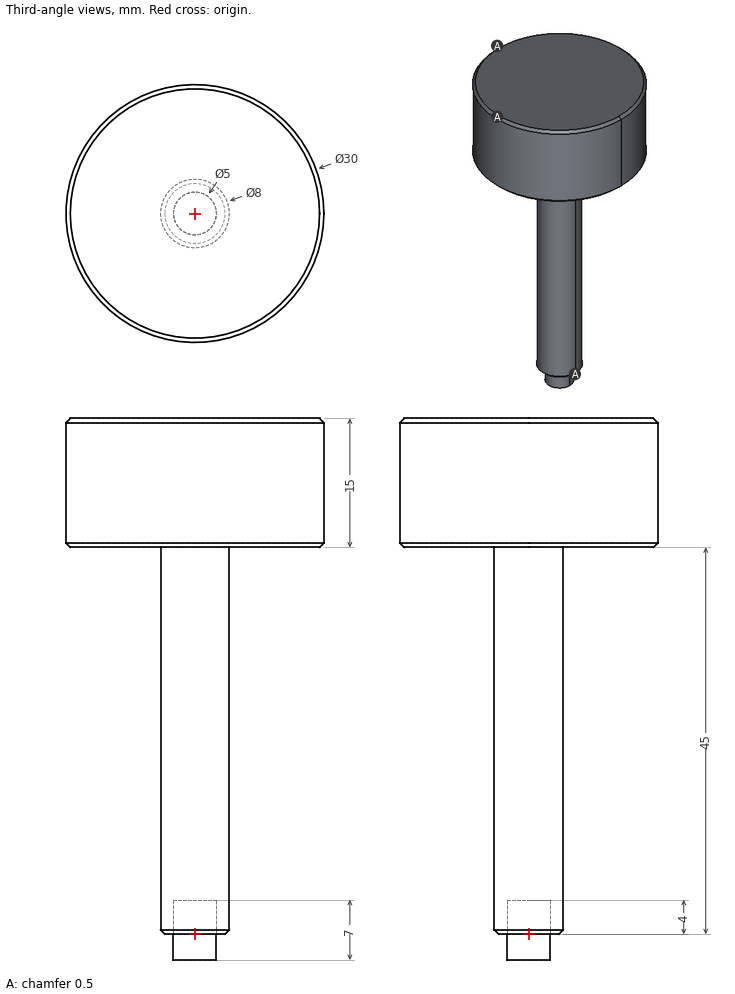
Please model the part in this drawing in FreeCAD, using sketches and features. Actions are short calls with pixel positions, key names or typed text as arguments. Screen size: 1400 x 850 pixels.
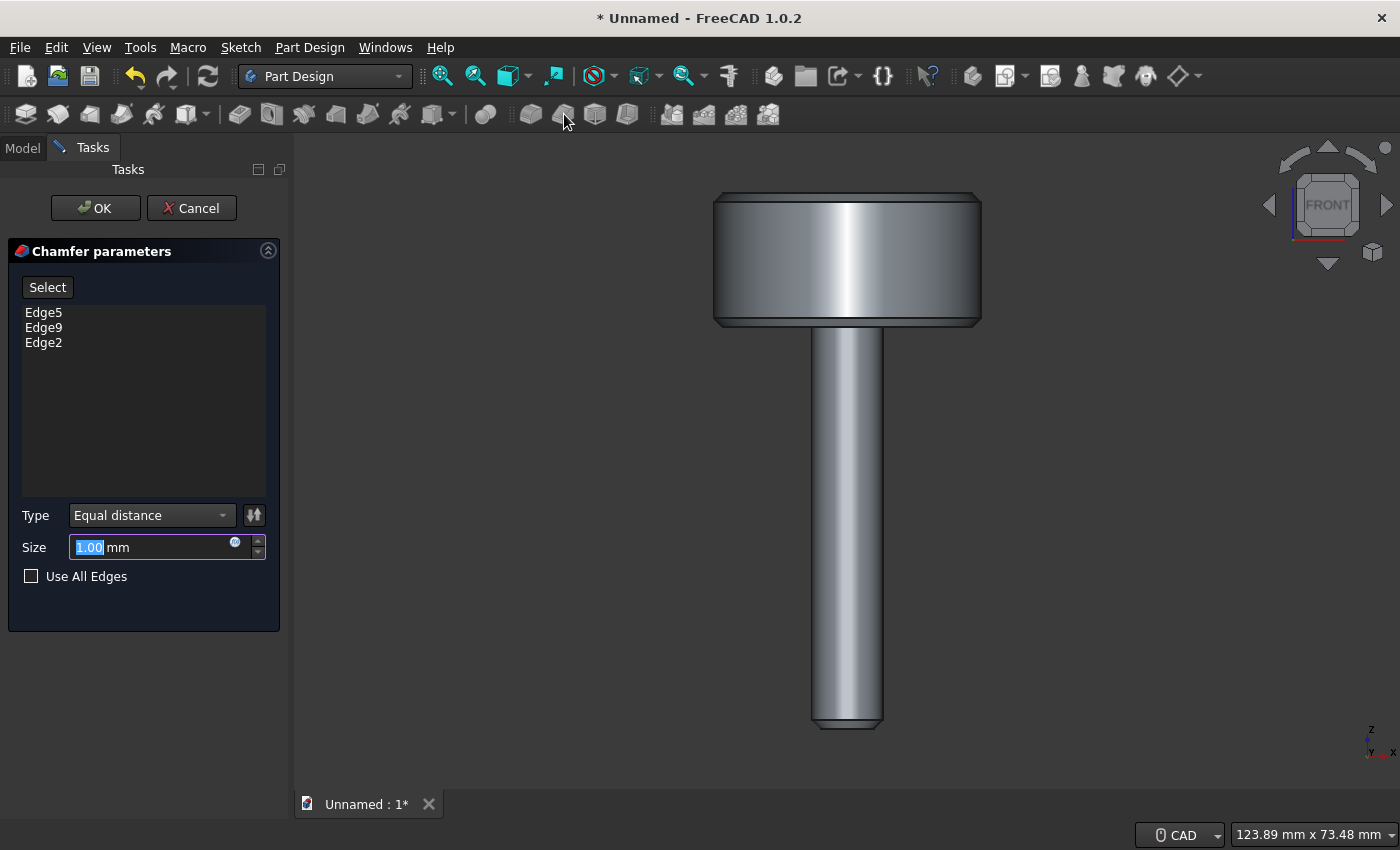
text(0.5)
key(Tab)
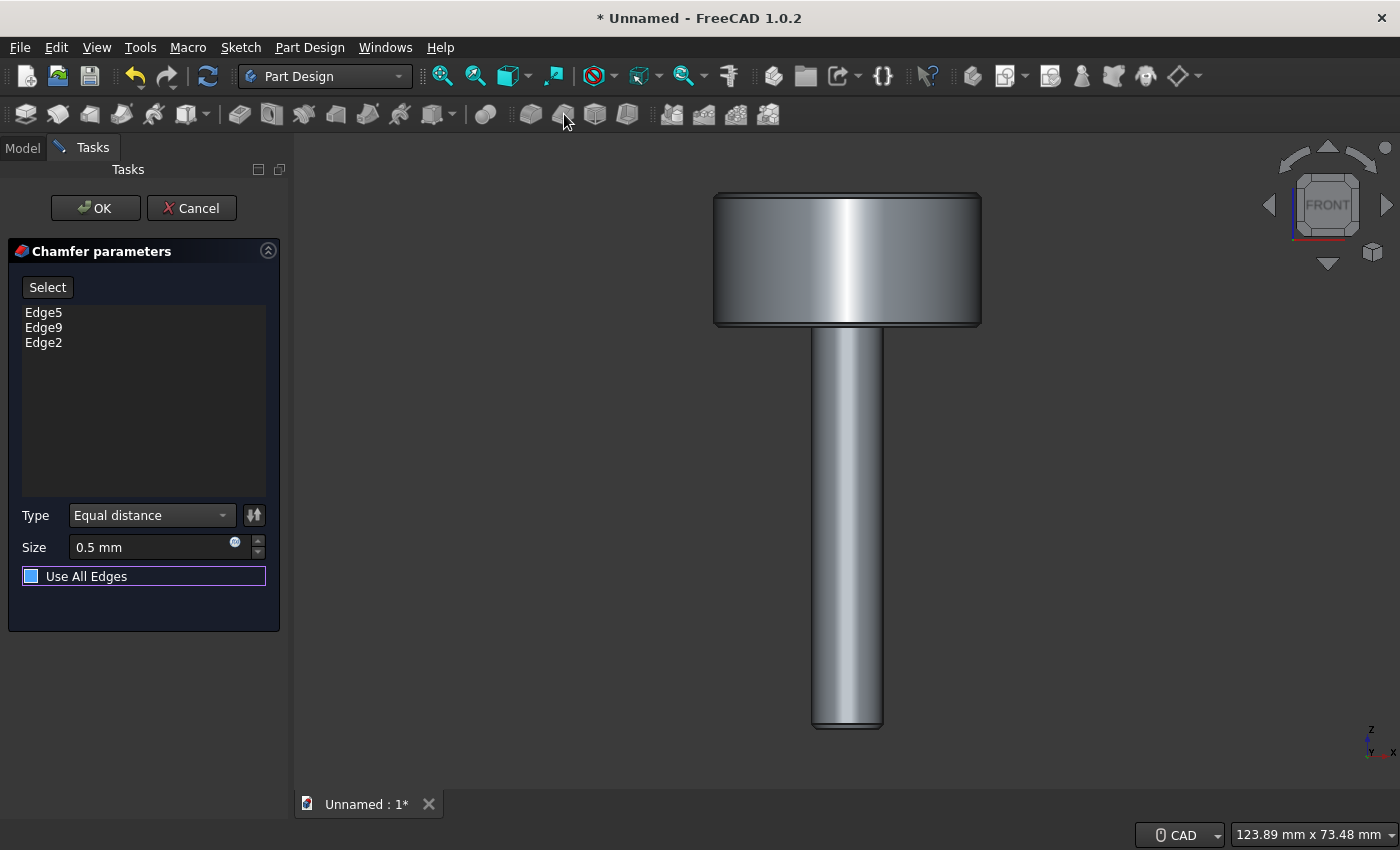
click(96, 208)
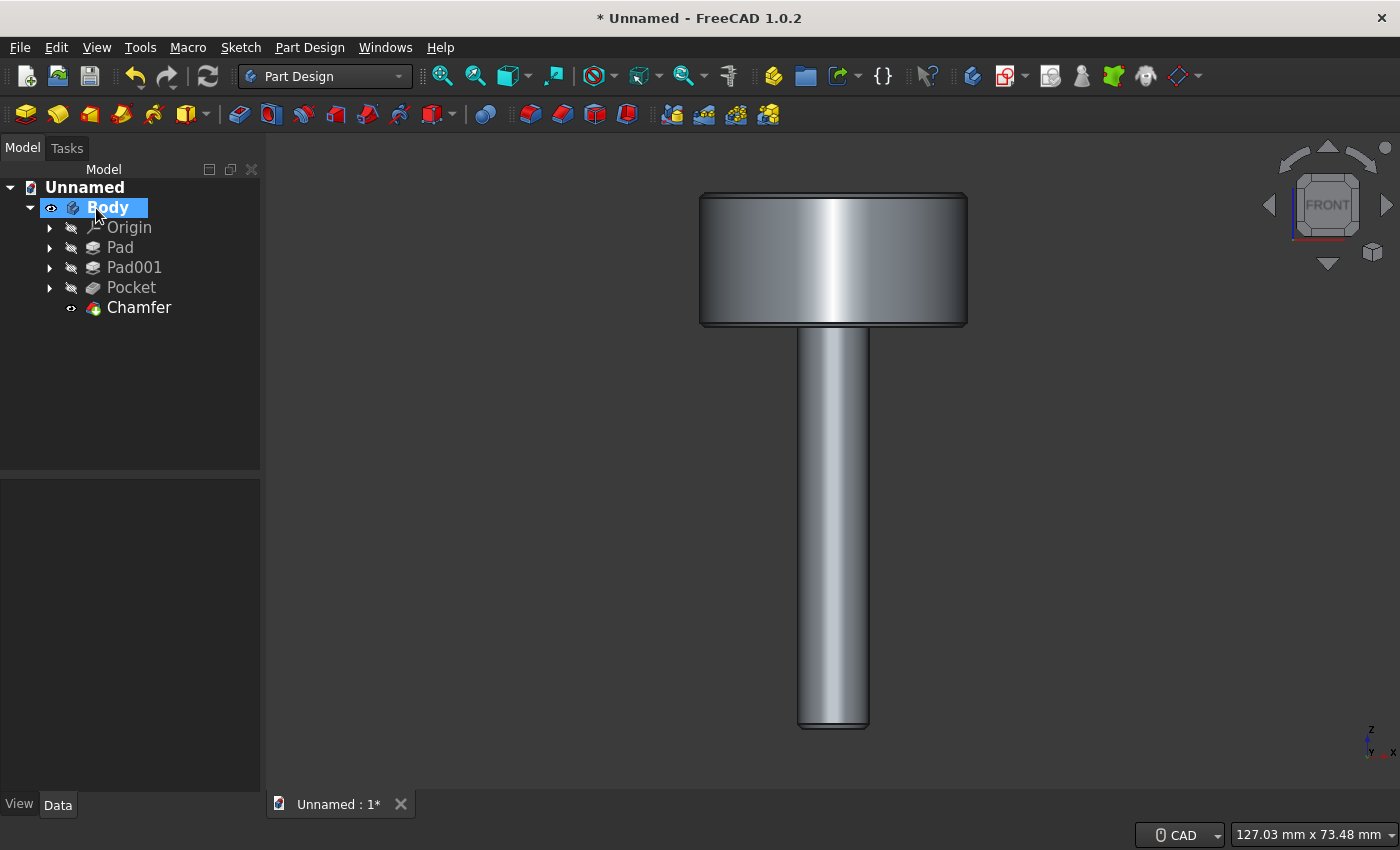
click(974, 76)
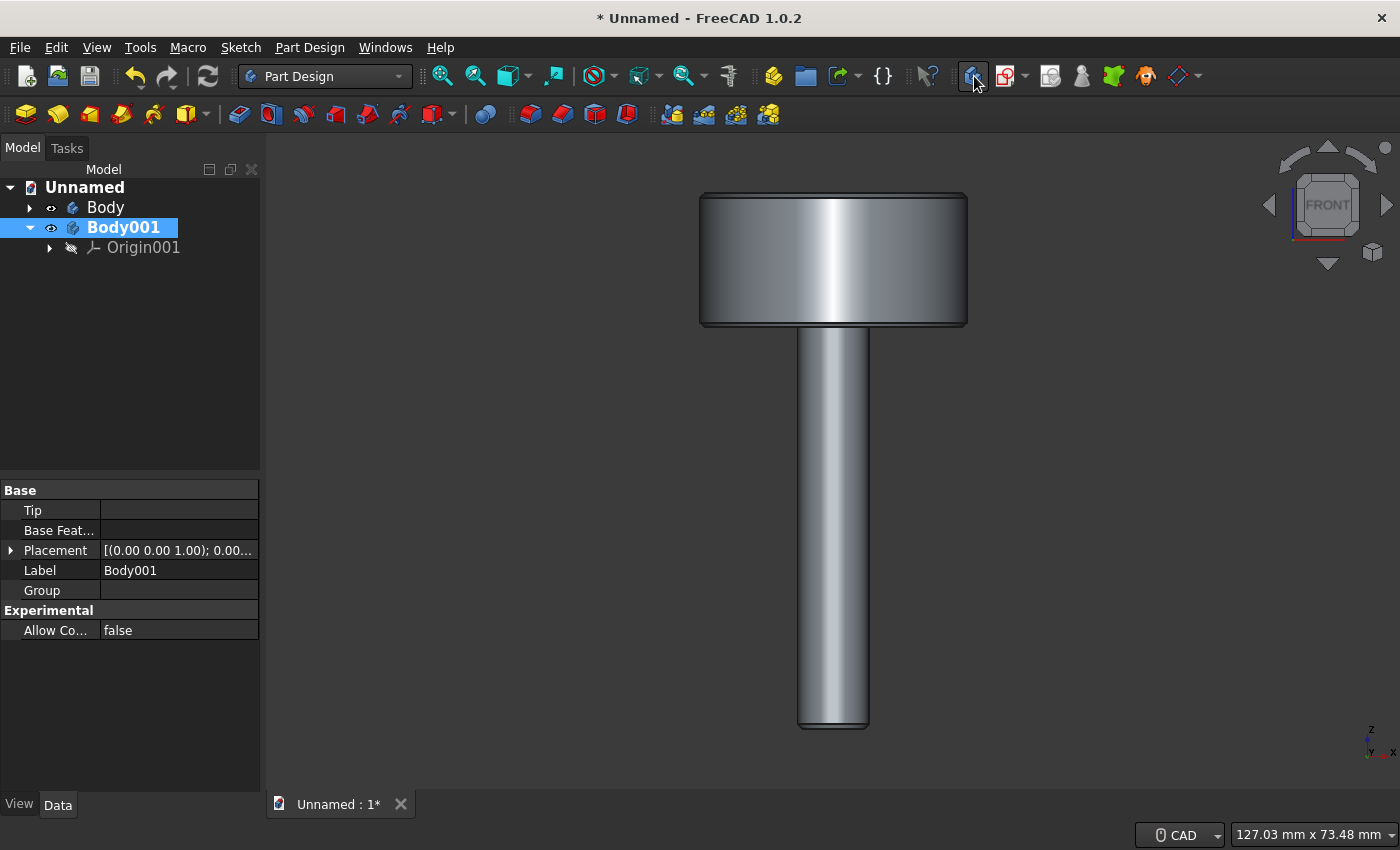
click(50, 248)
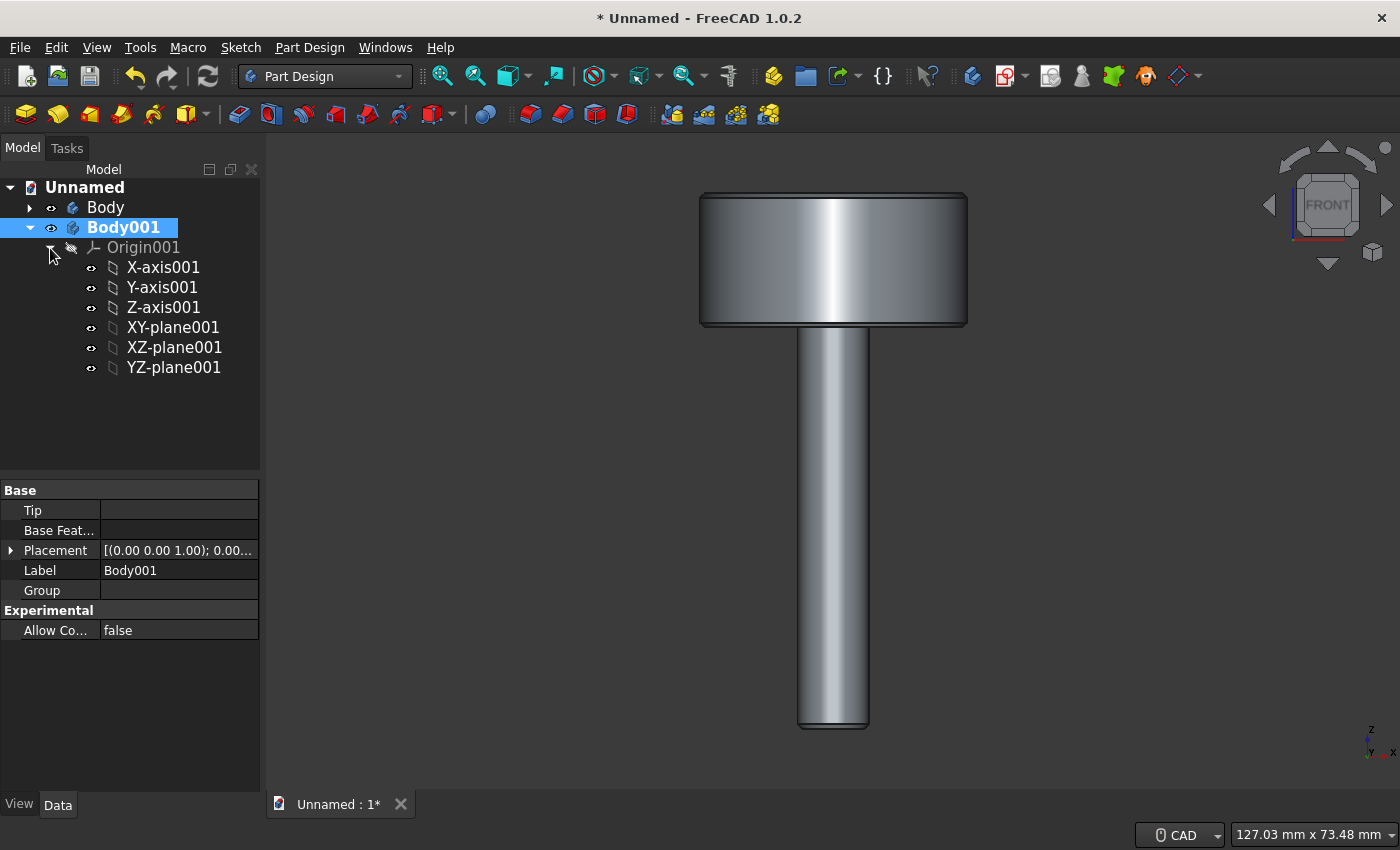
click(136, 328)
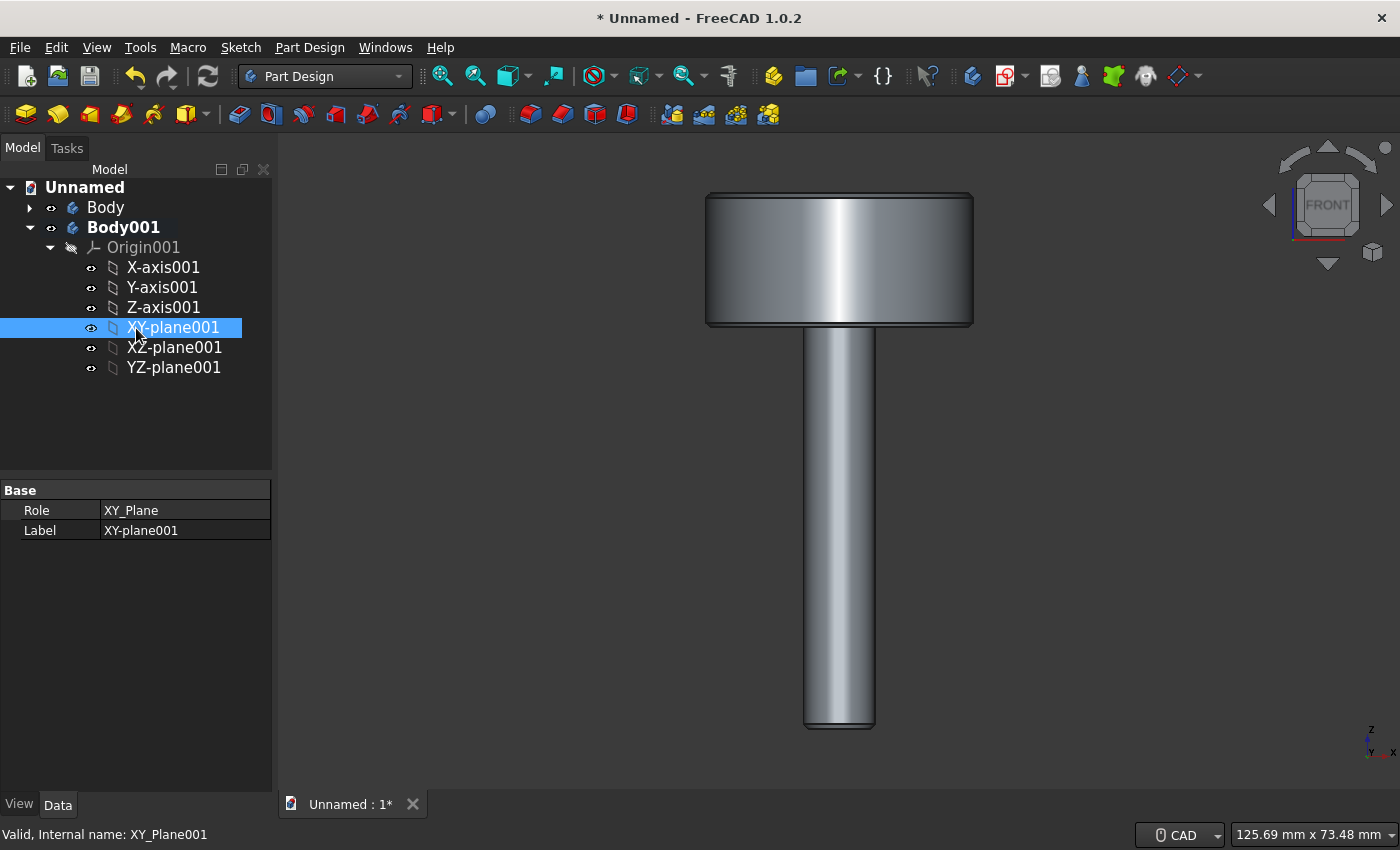
click(1178, 76)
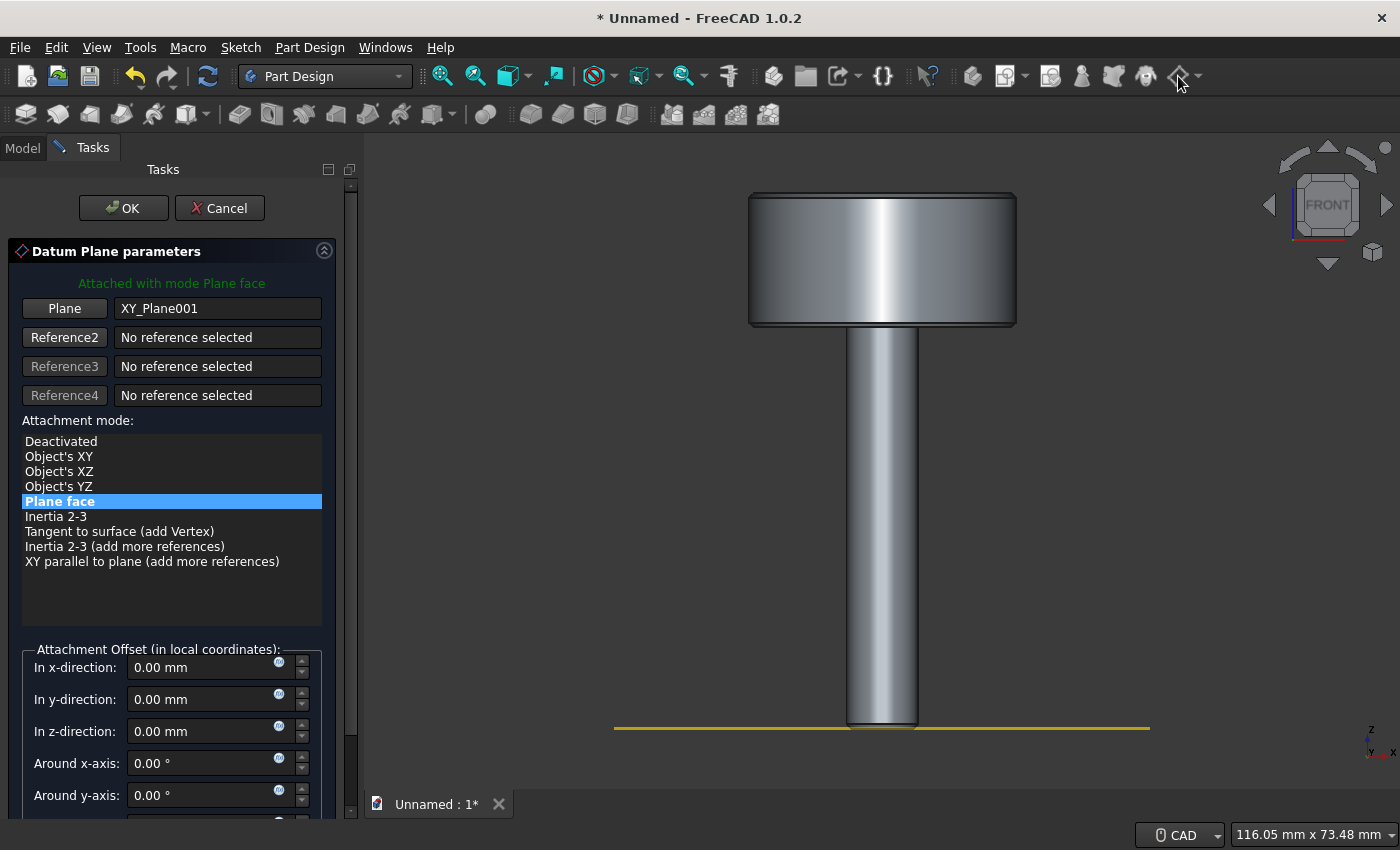
triple_click(210, 731)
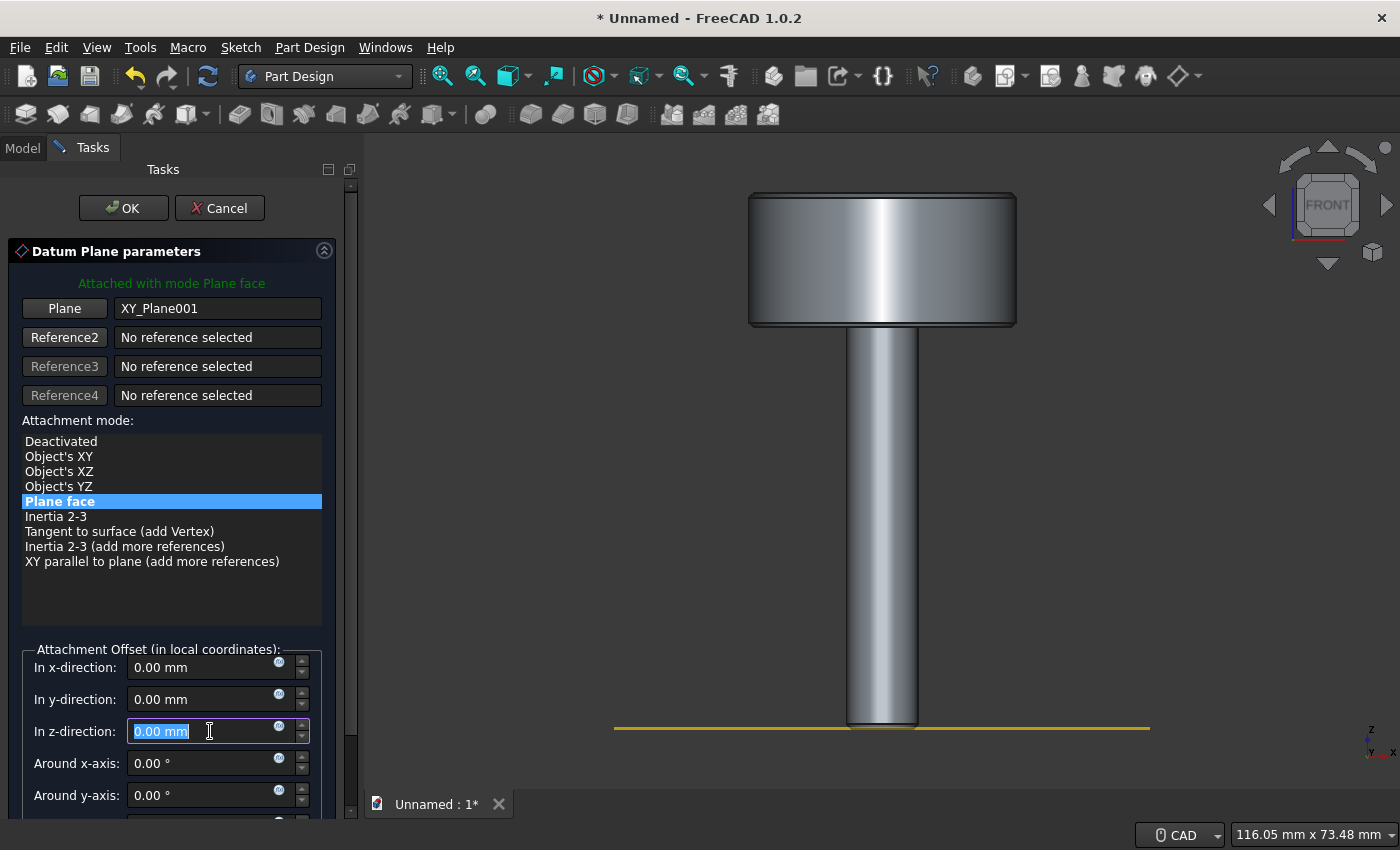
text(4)
key(Tab)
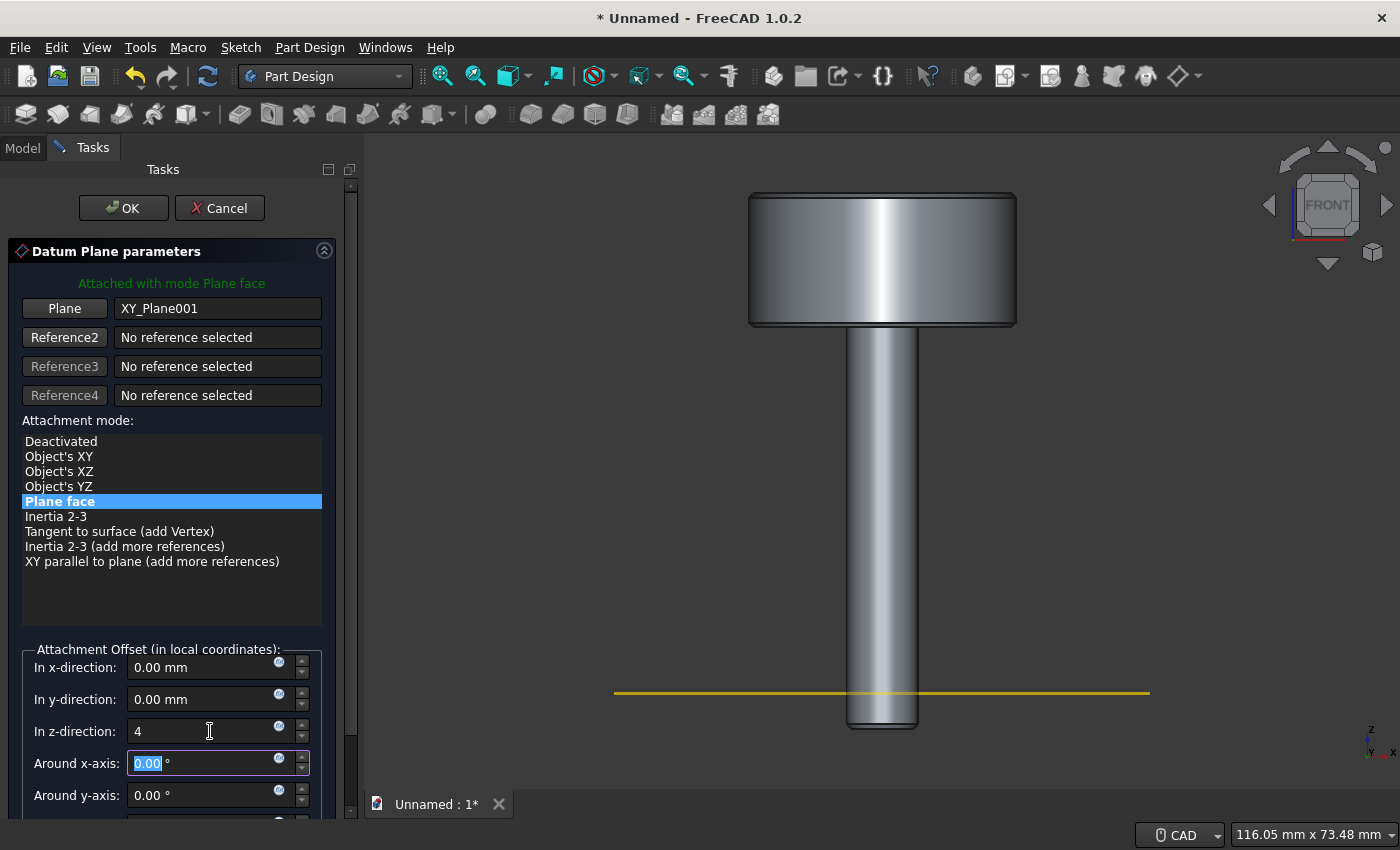
click(124, 208)